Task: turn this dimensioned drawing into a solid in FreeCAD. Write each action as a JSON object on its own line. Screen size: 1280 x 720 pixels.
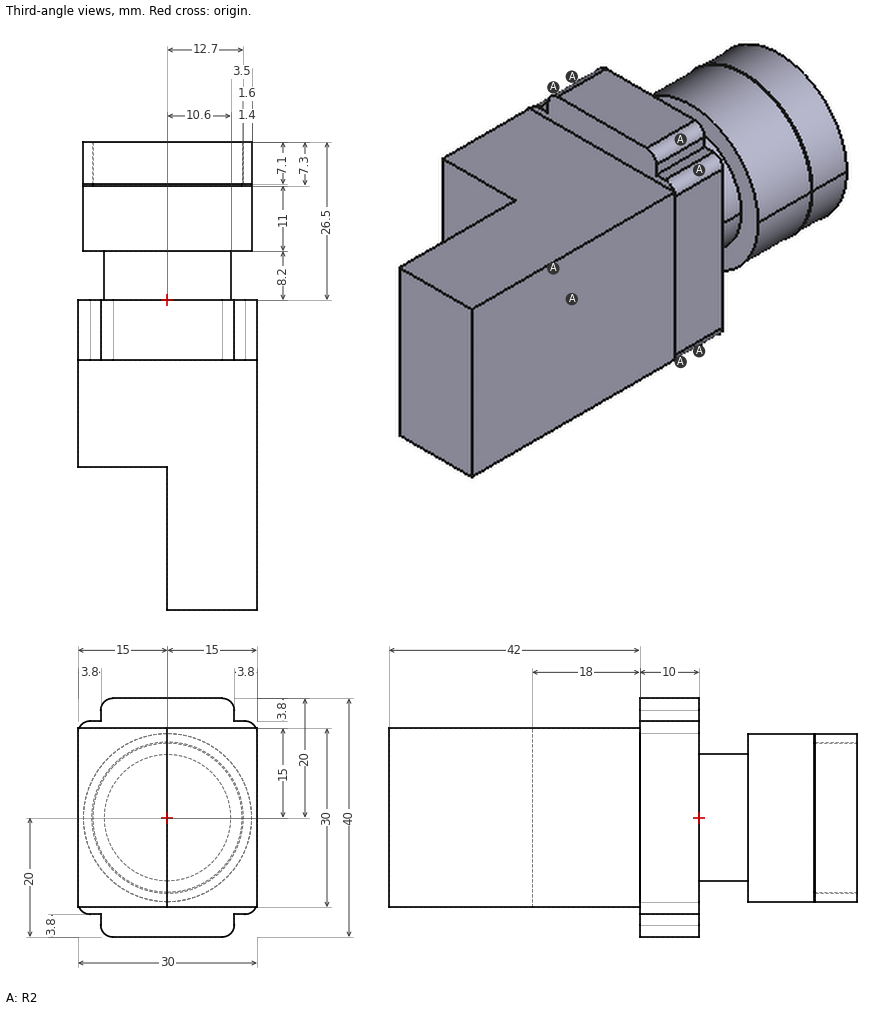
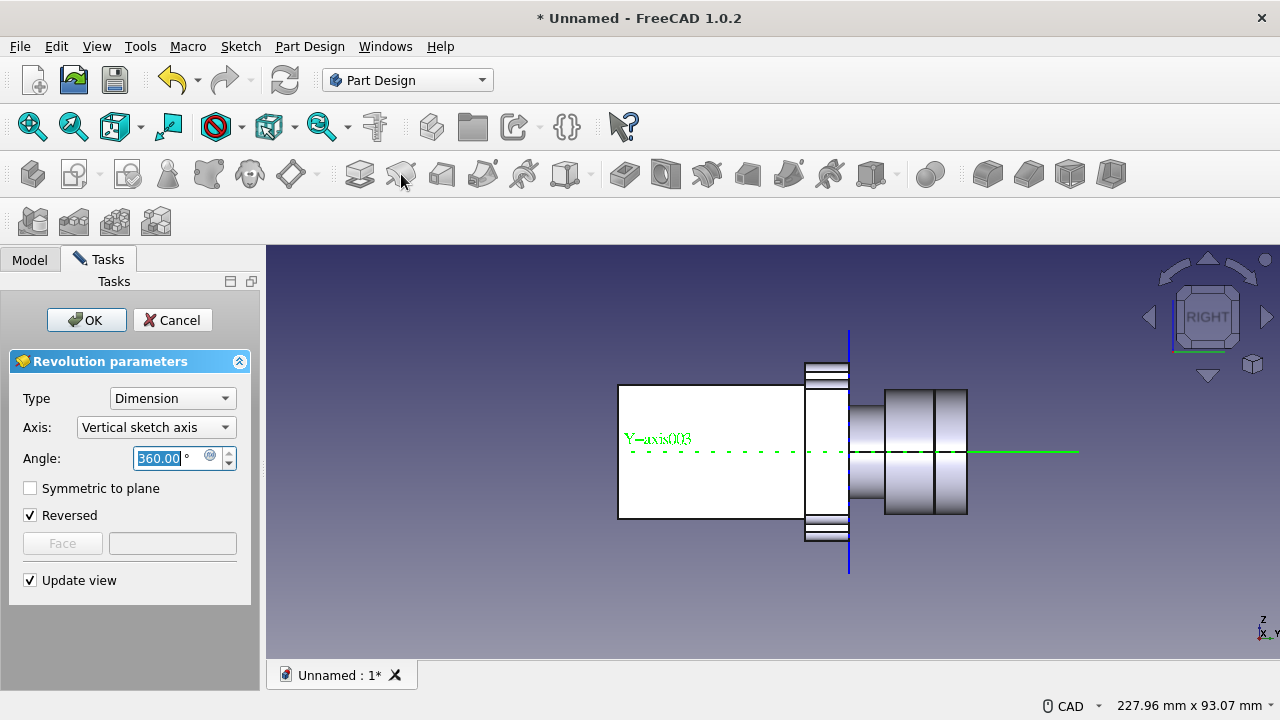
{"action": "left_click", "coordinate": [87, 320]}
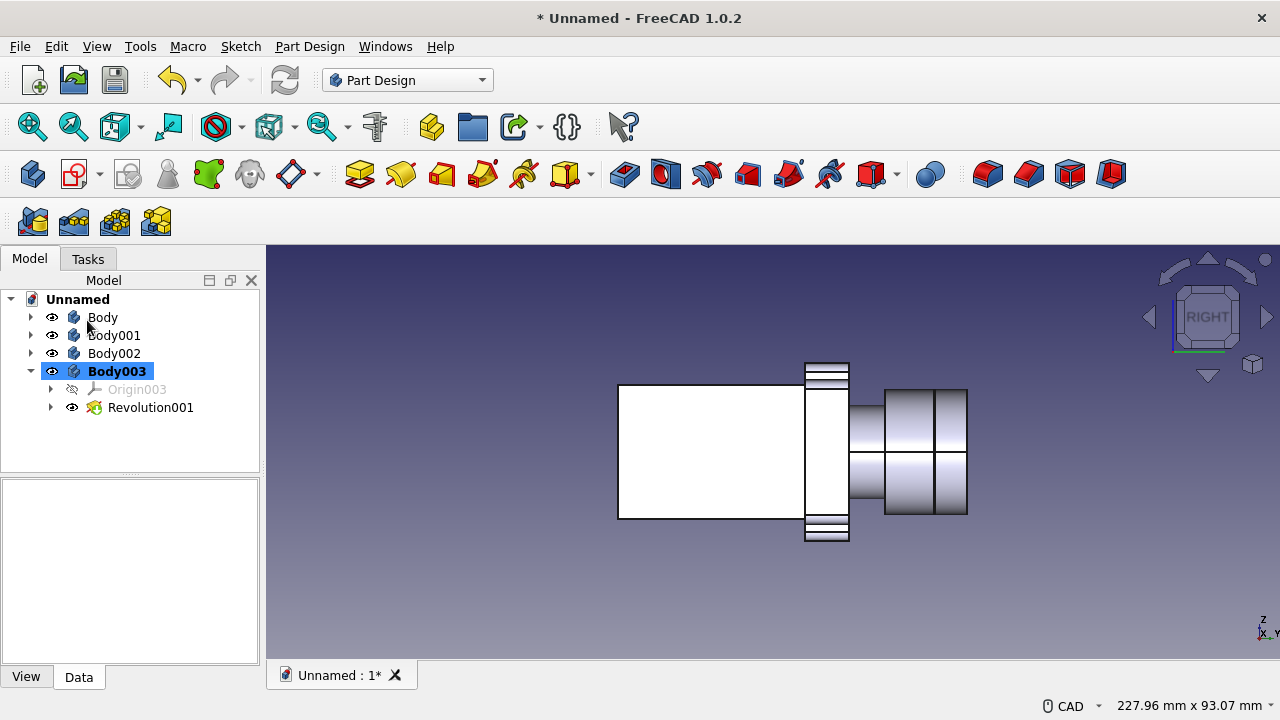
{"action": "key", "text": "0"}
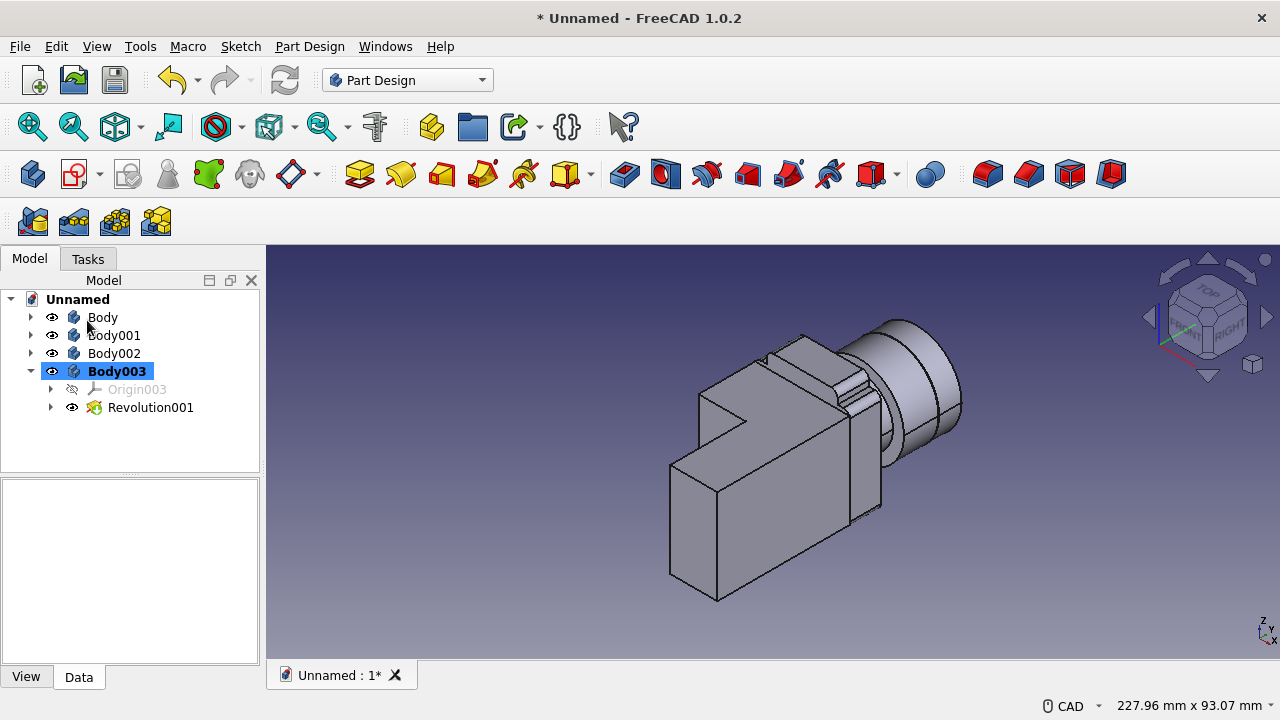
{"action": "left_click", "coordinate": [33, 128]}